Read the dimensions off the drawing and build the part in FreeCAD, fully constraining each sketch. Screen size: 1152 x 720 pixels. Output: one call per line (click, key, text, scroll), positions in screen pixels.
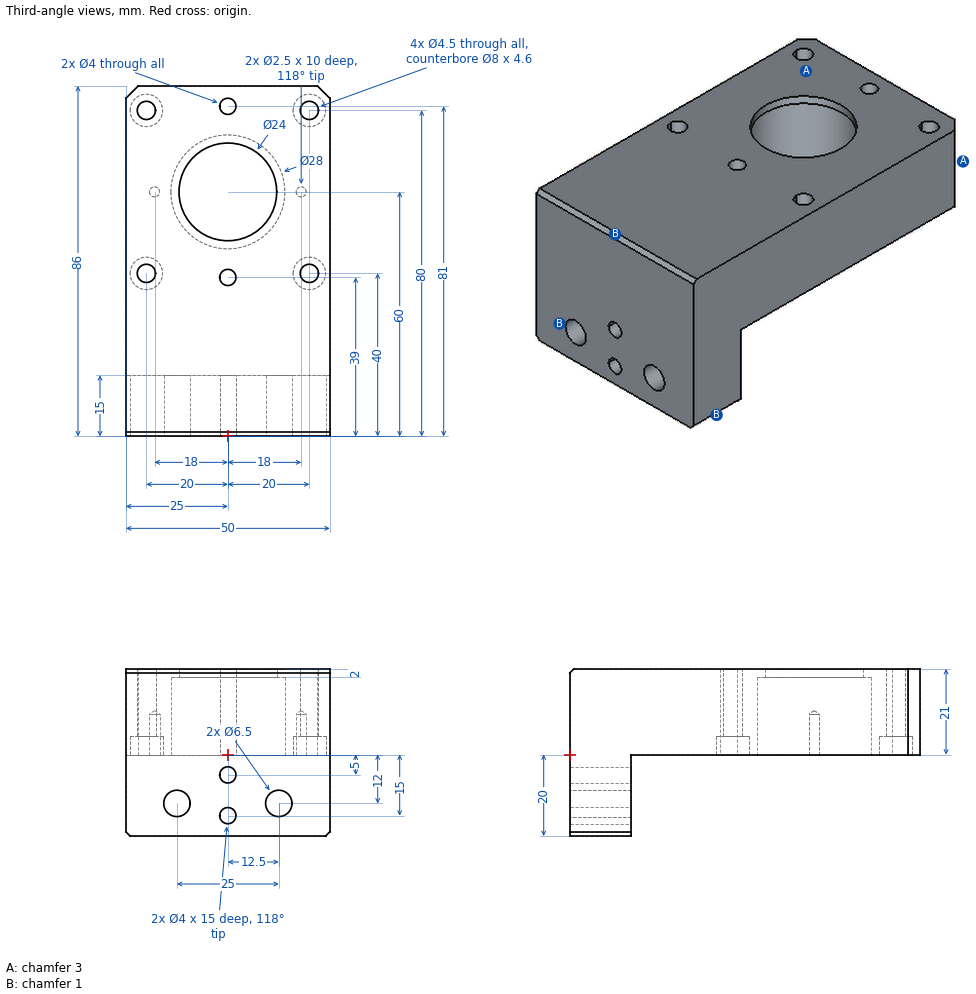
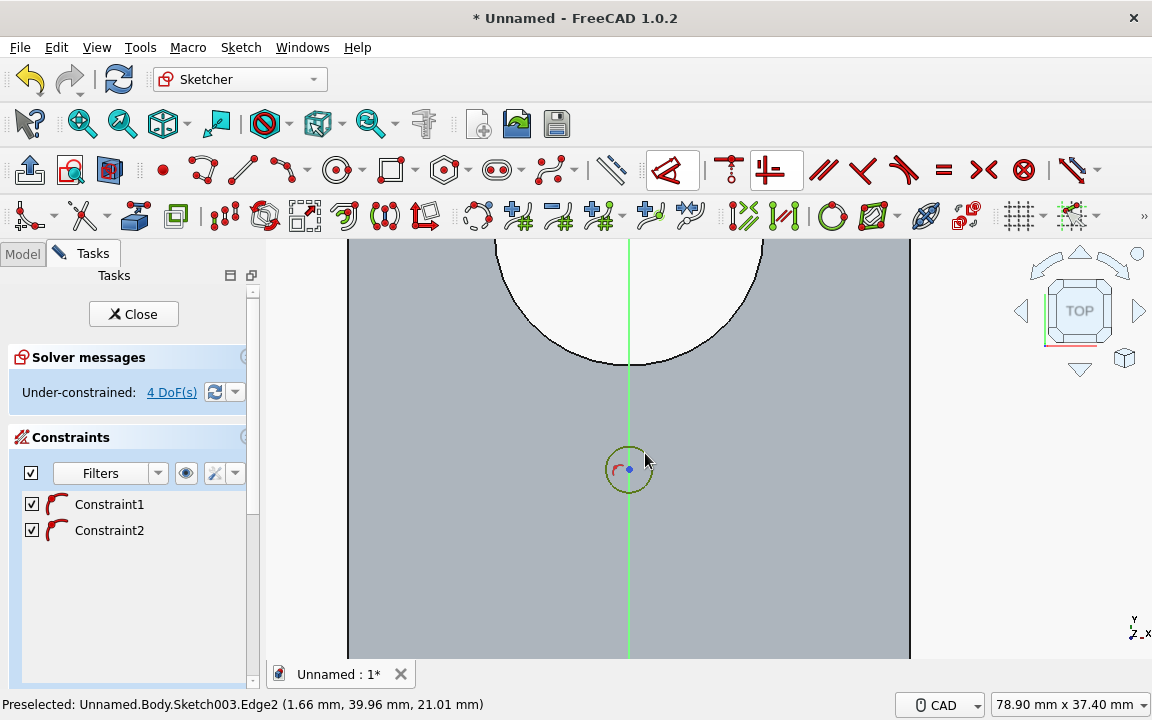
click(944, 170)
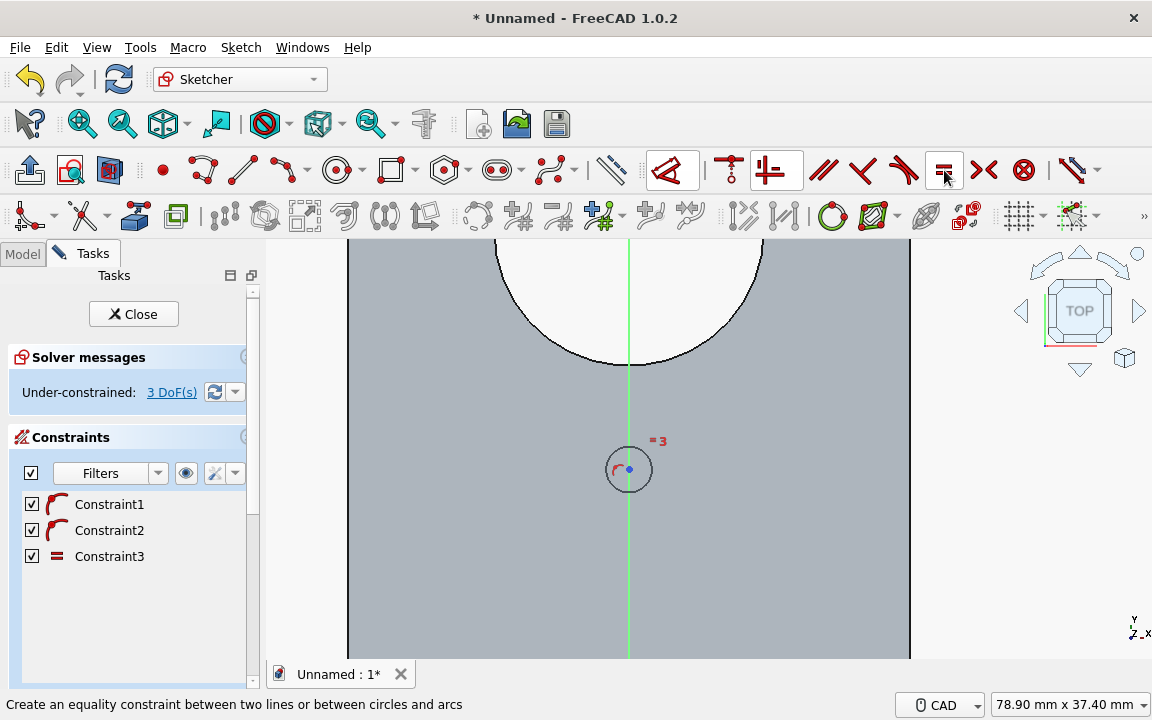
scroll(645, 453, down, 6)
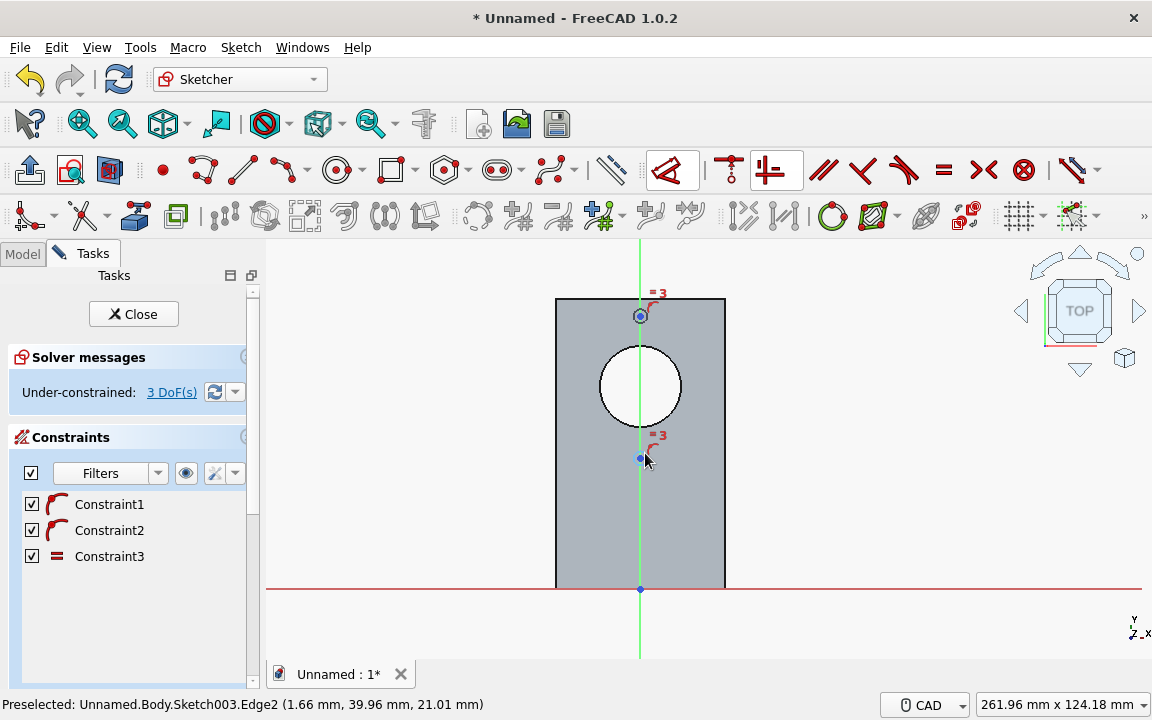
scroll(645, 311, up, 6)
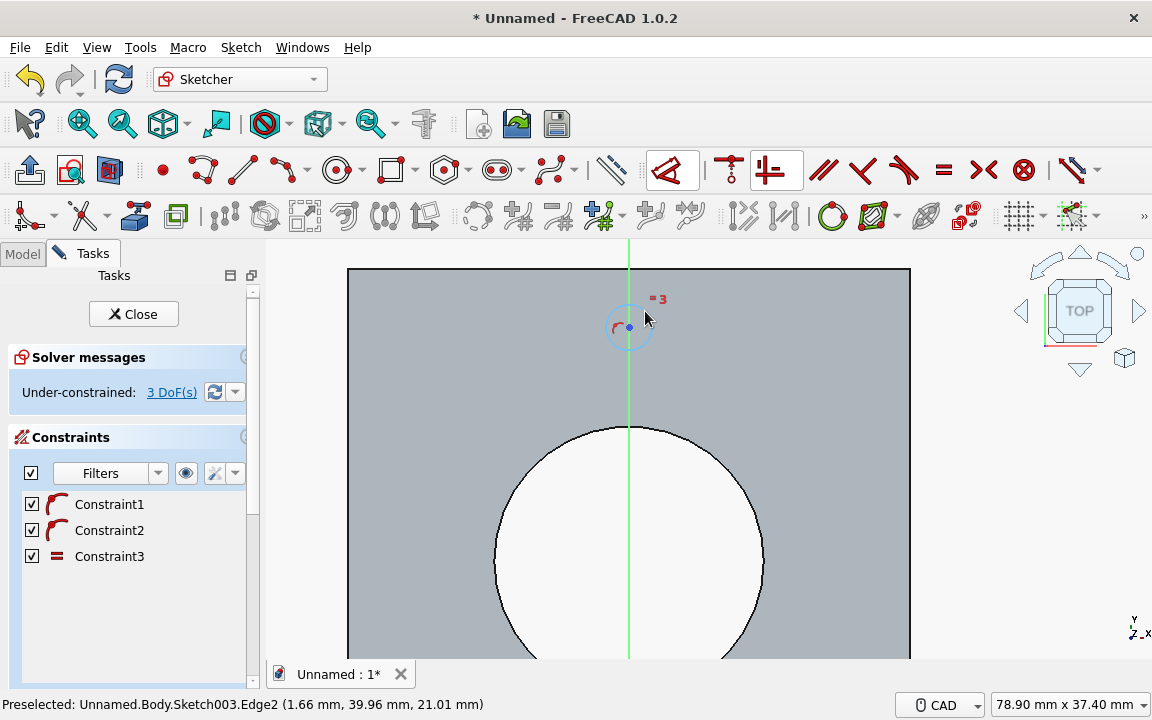
click(645, 311)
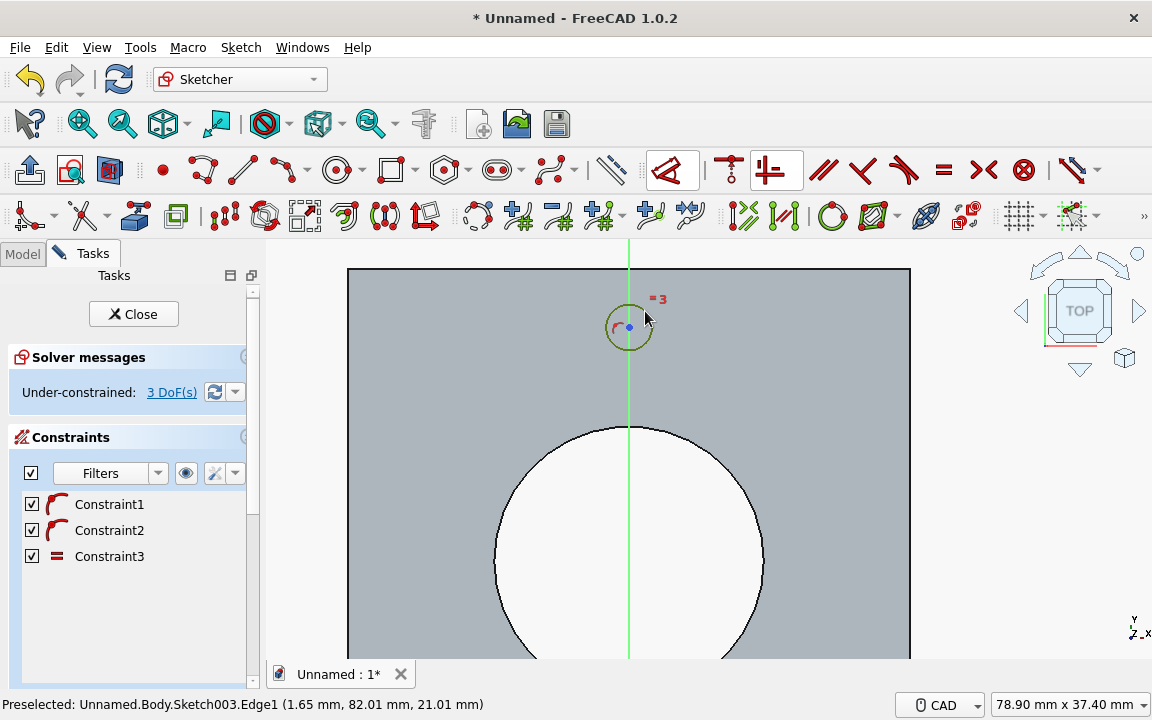
click(694, 170)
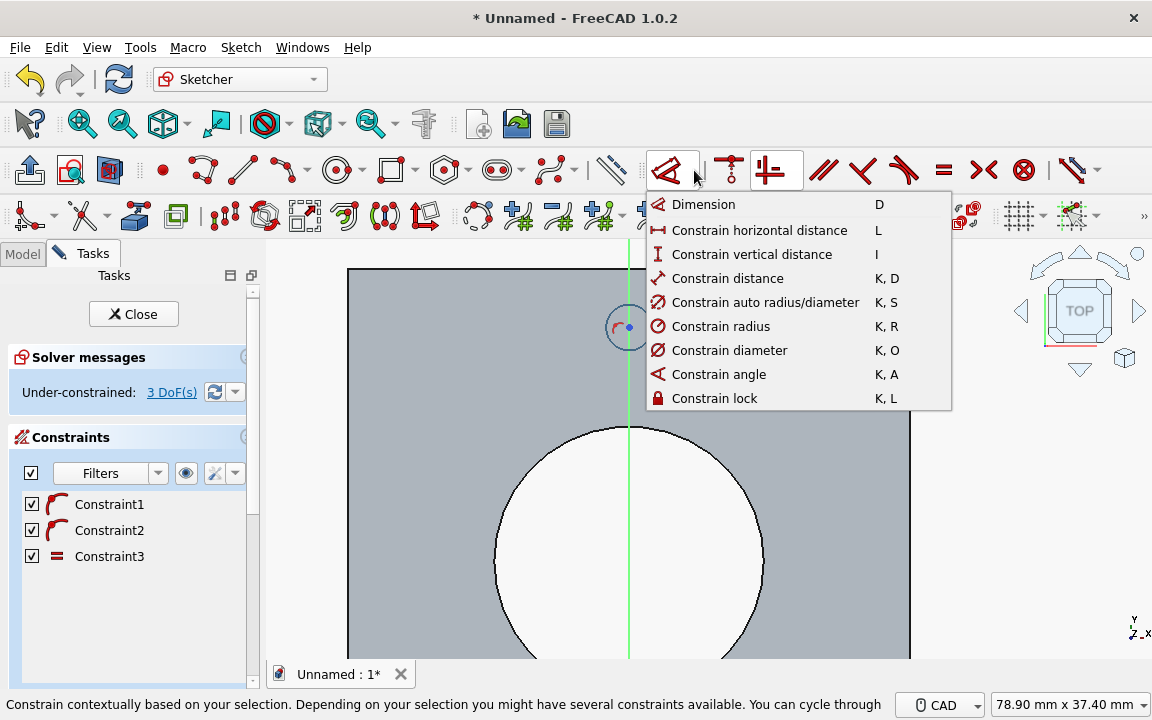
click(799, 350)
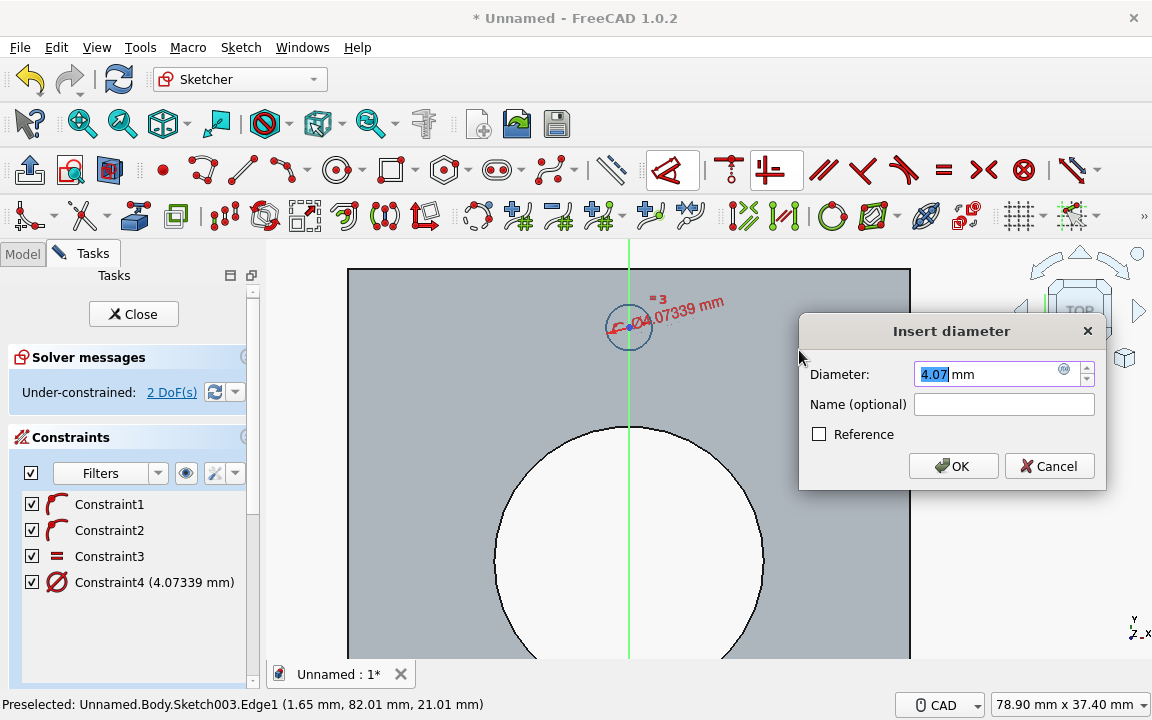
text(4)
key(Return)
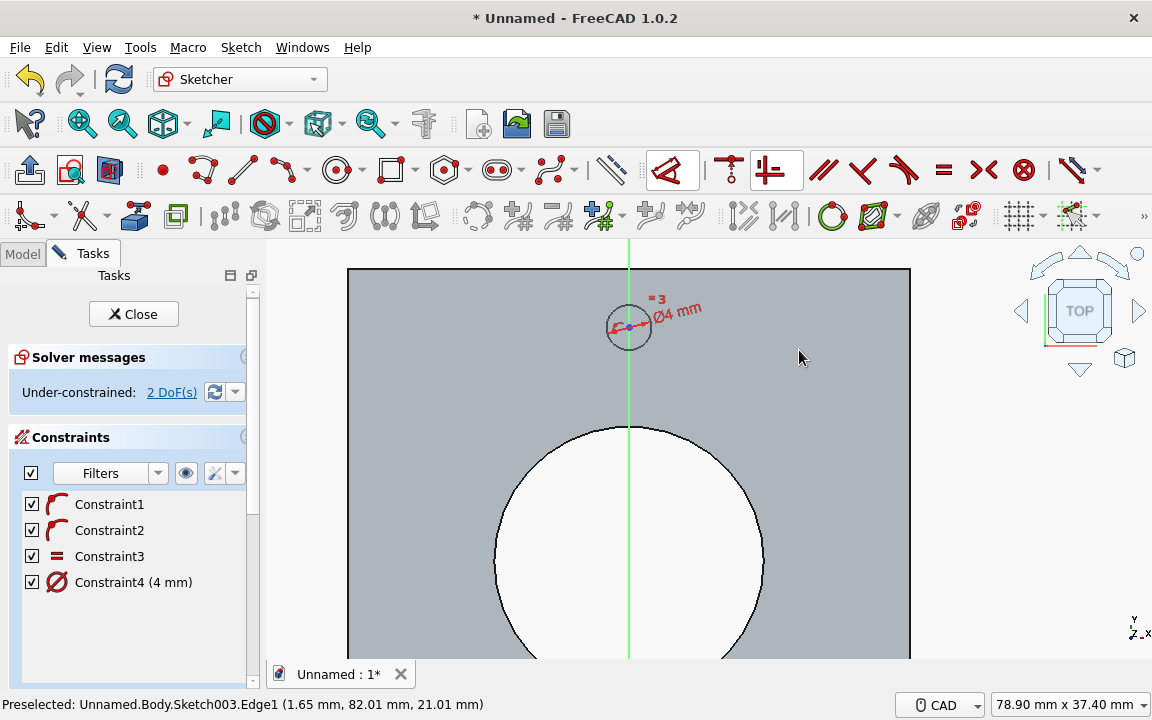
click(629, 328)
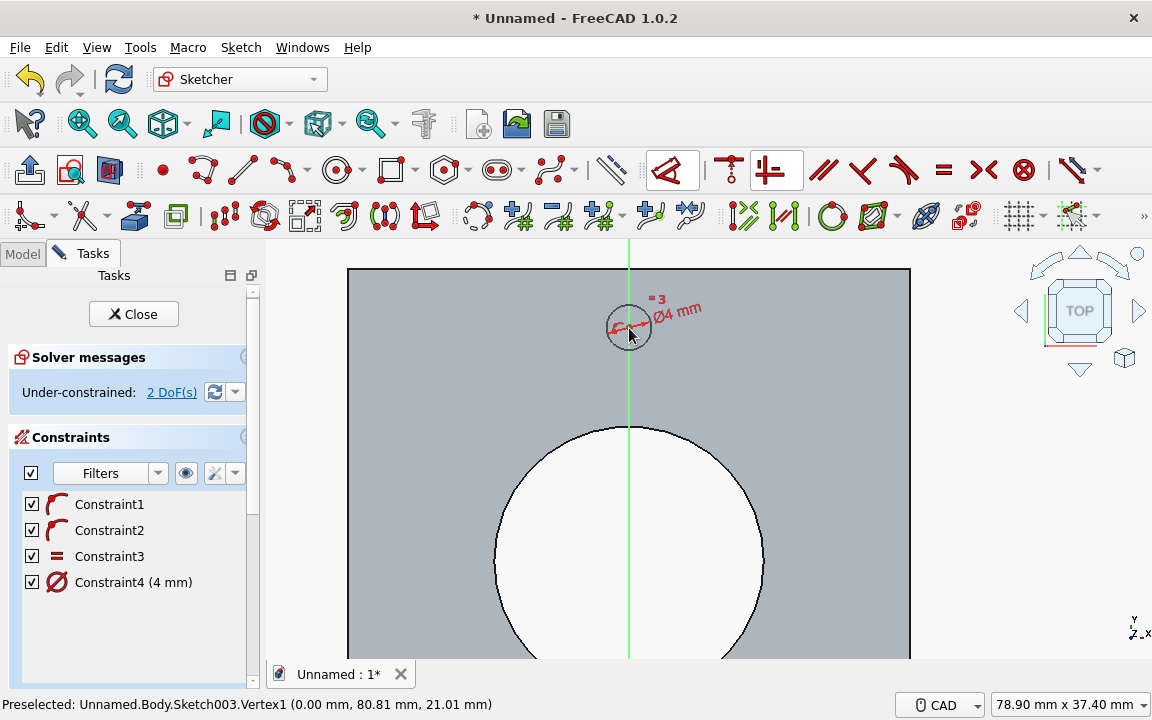
key(i)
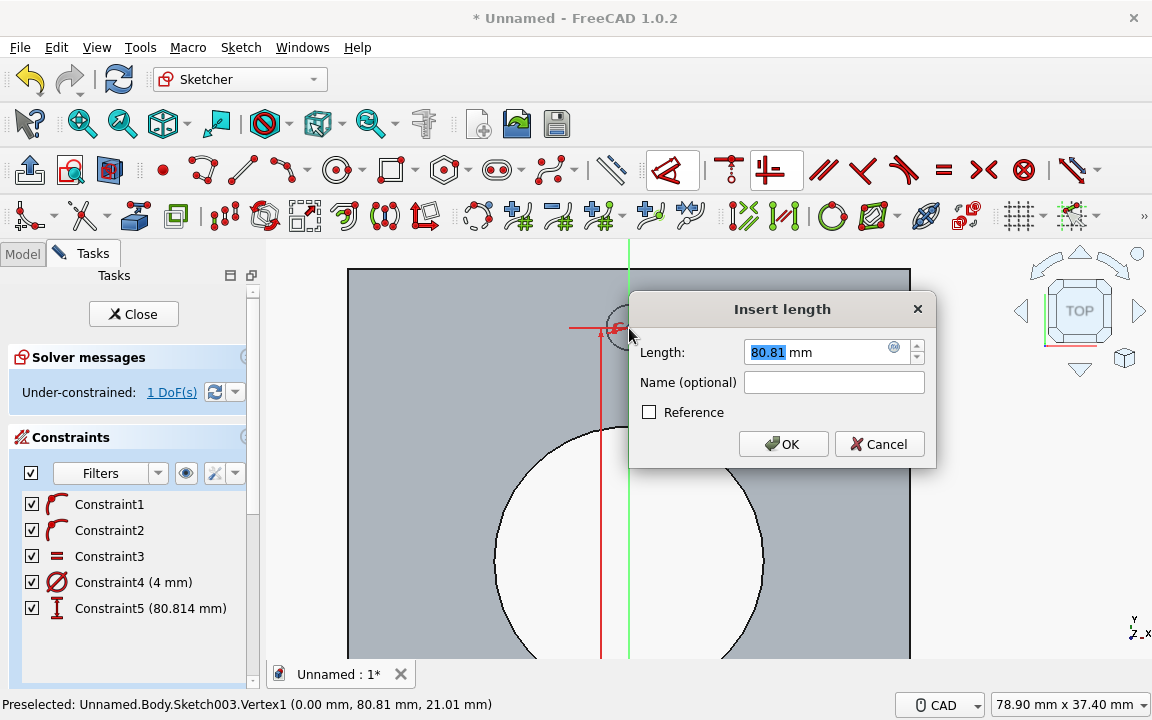
text(81)
key(Return)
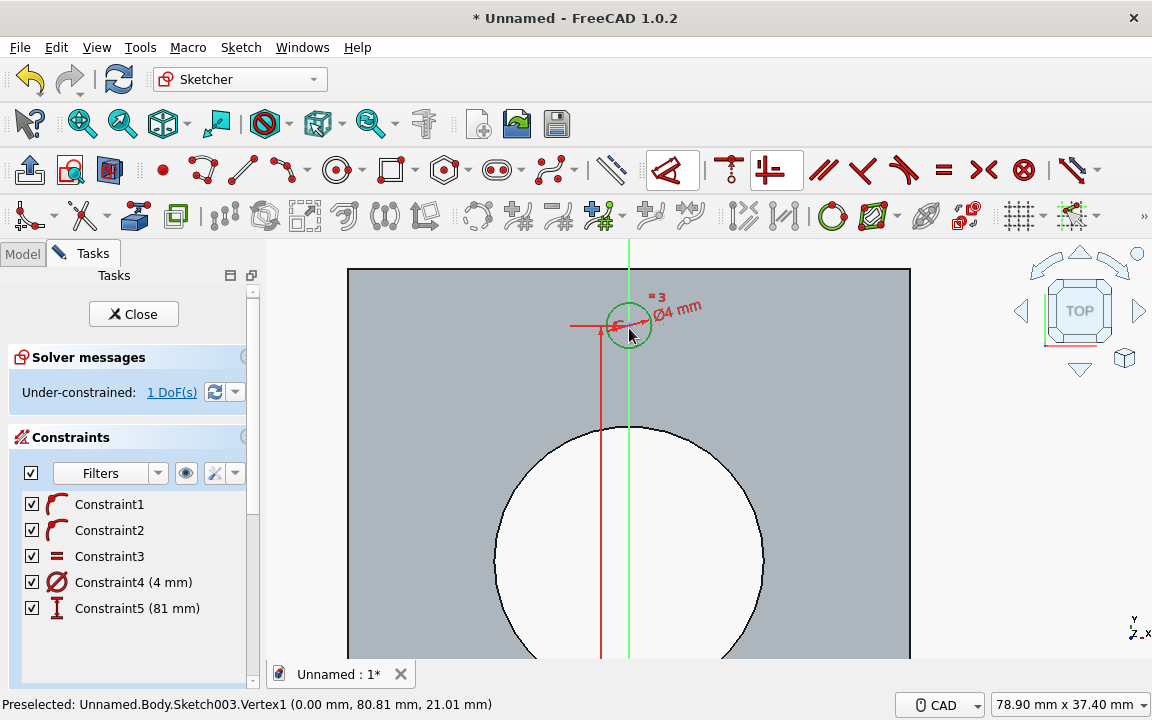
scroll(645, 311, down, 6)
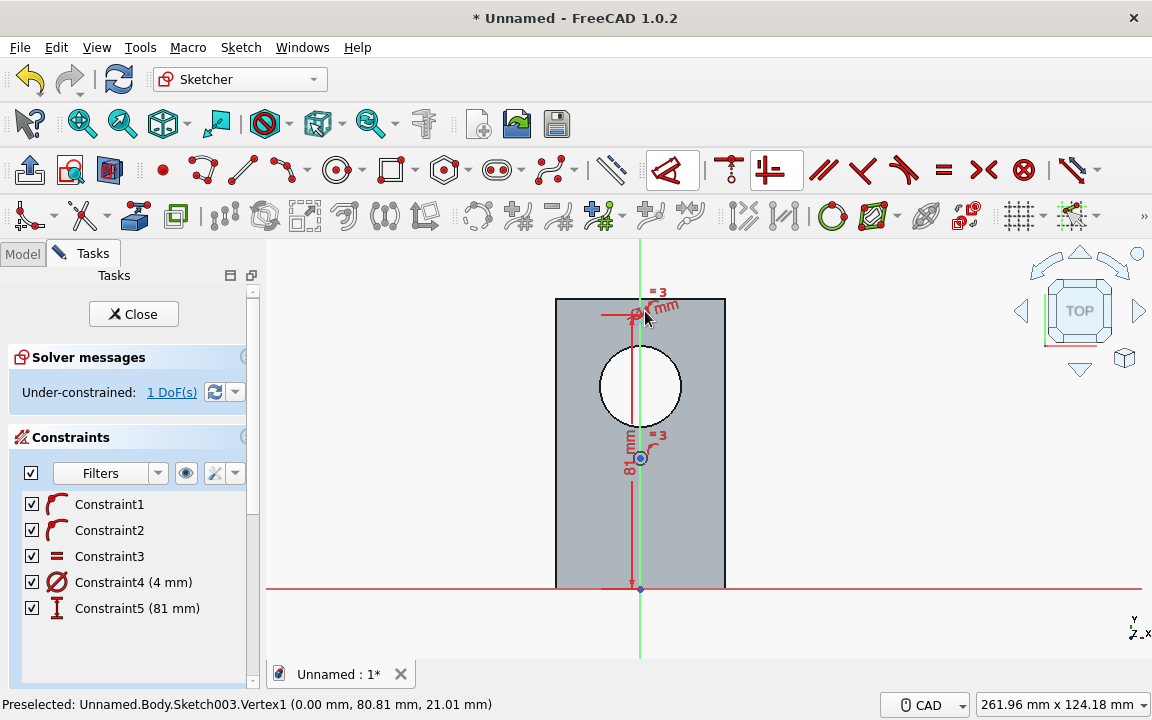
click(640, 458)